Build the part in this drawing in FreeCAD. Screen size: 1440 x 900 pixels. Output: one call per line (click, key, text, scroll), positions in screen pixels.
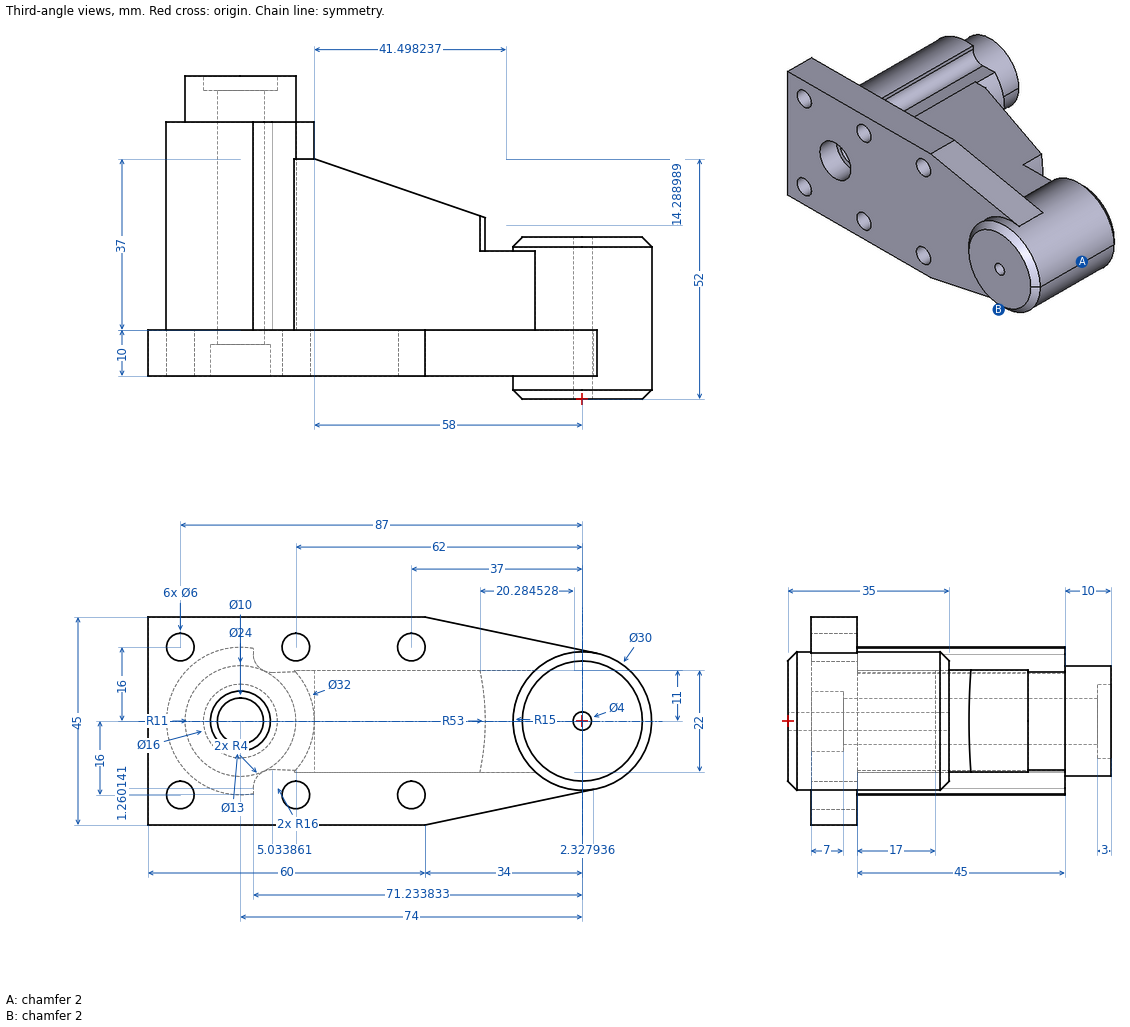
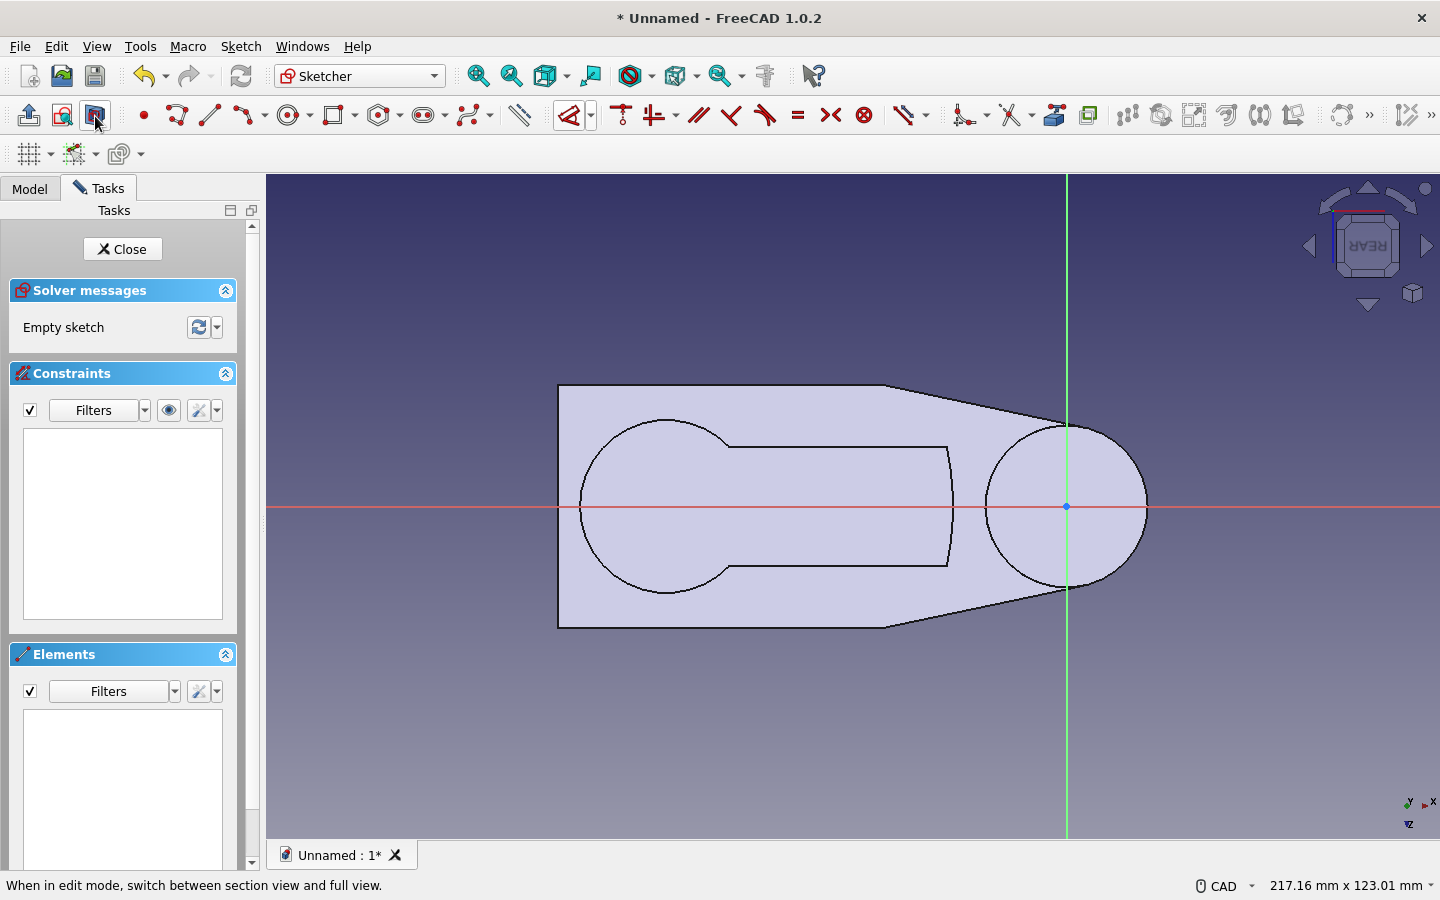
scroll(1102, 506, up, 6)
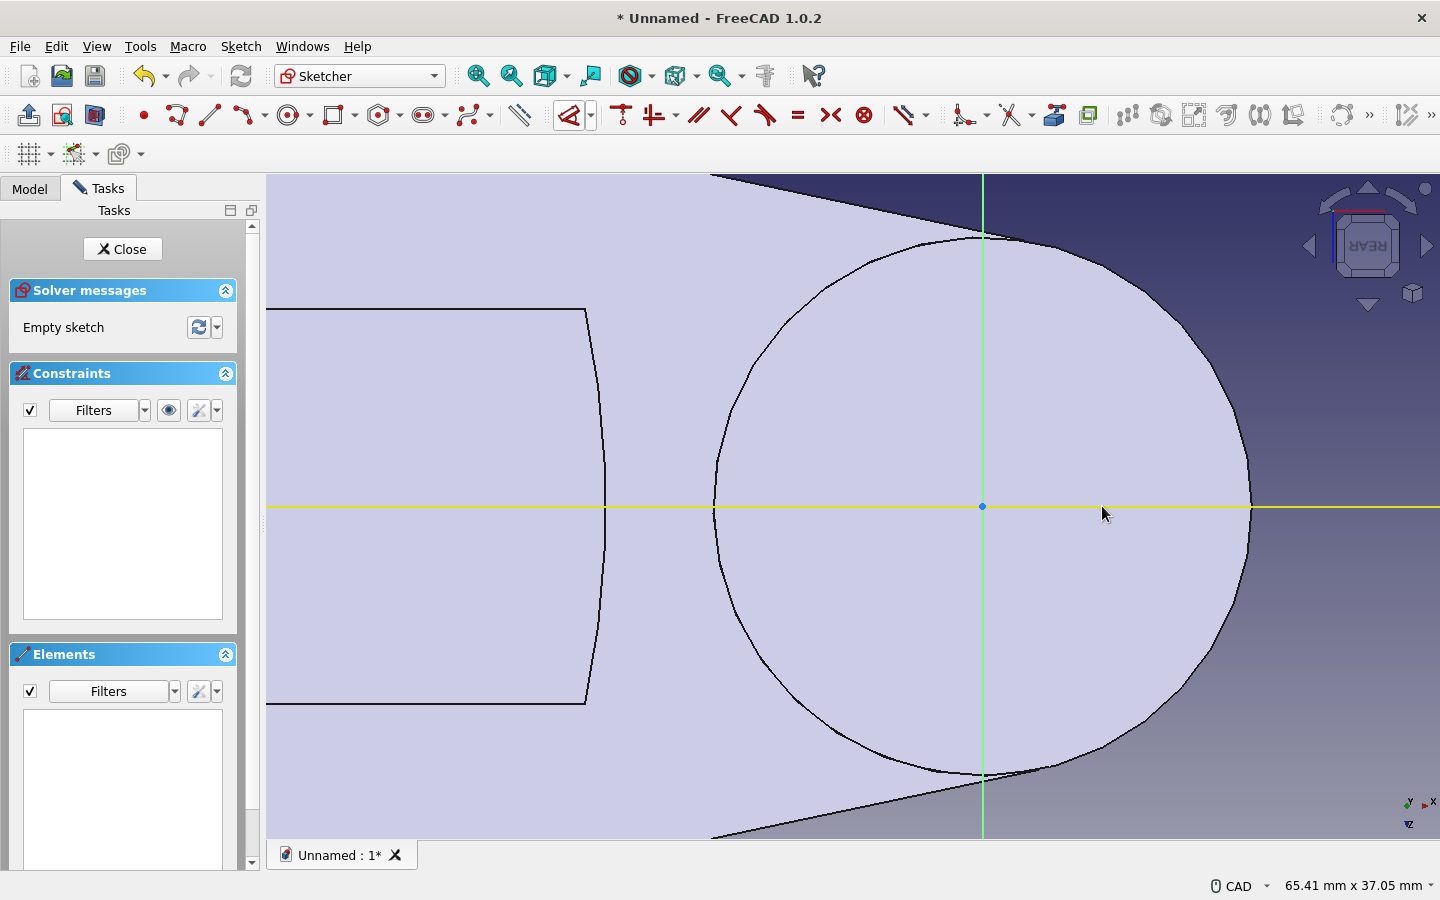
click(177, 116)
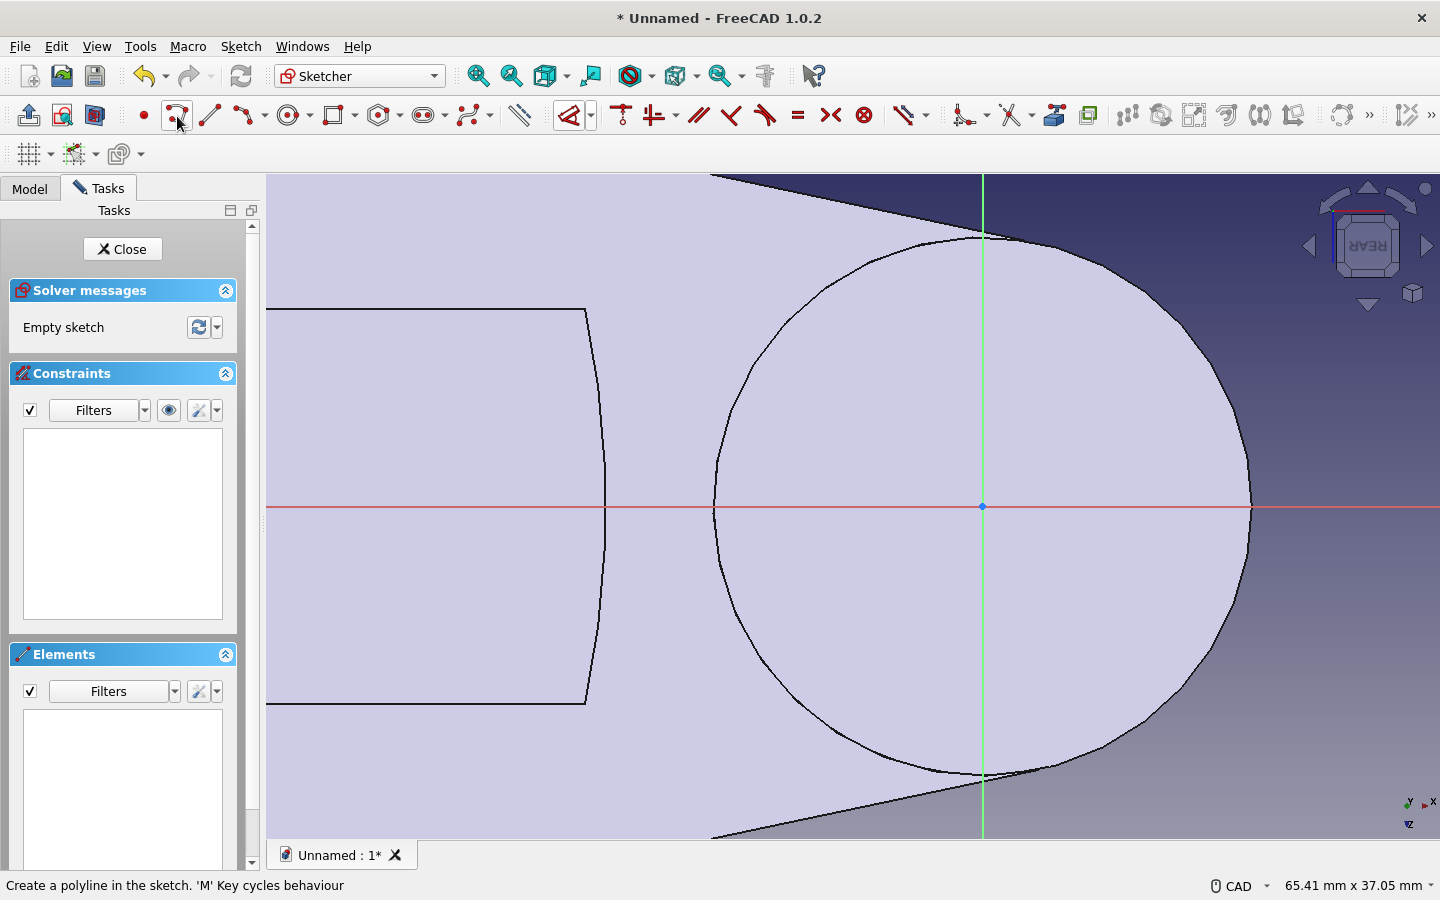
click(585, 704)
click(949, 704)
click(949, 309)
click(585, 309)
right_click(585, 309)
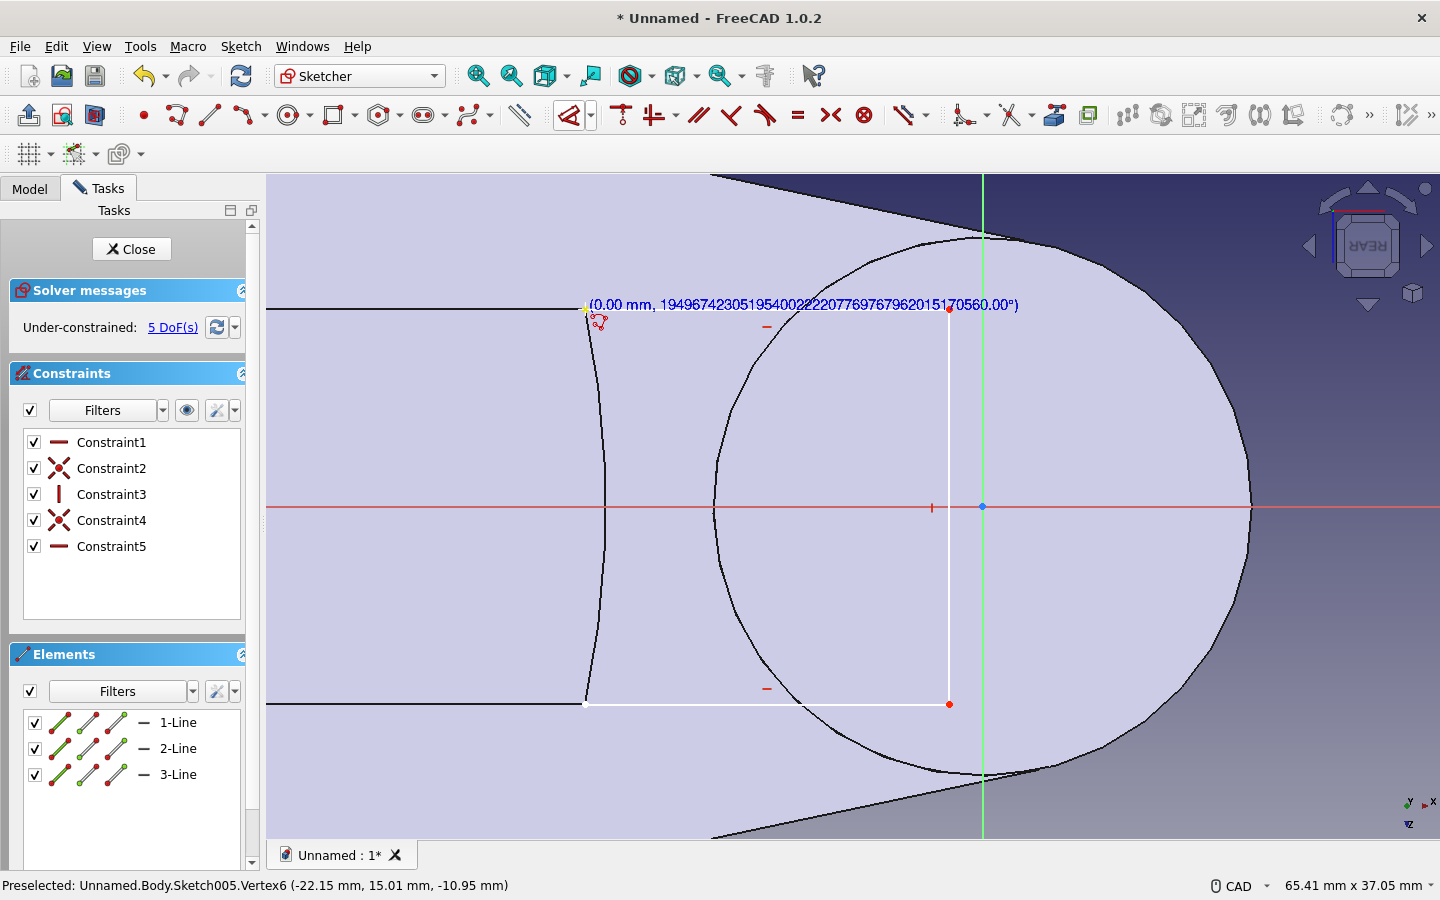
click(242, 116)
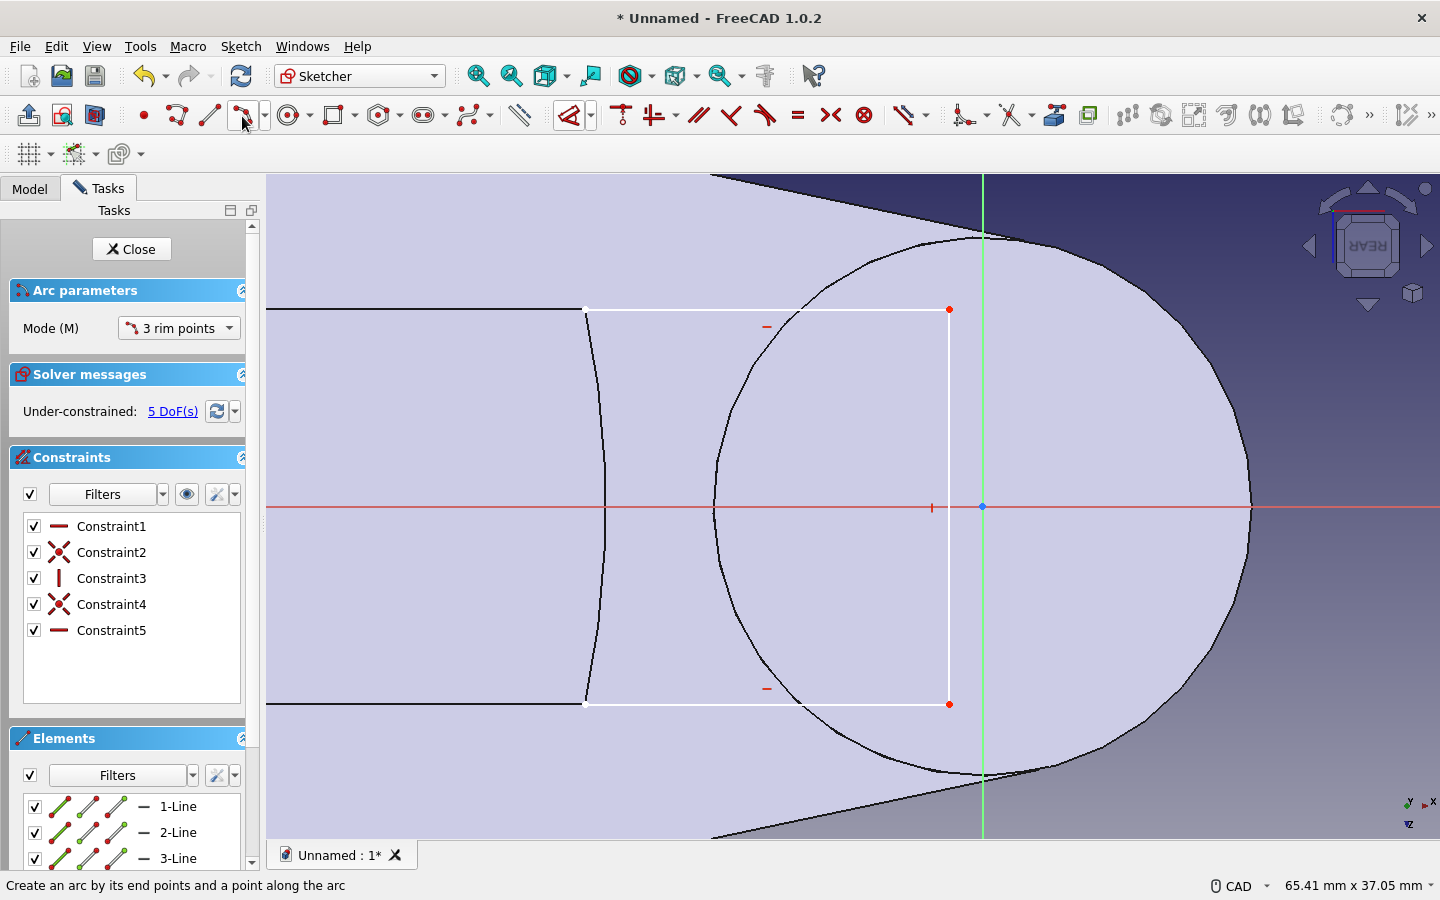
click(585, 310)
click(585, 705)
click(605, 546)
key(Escape)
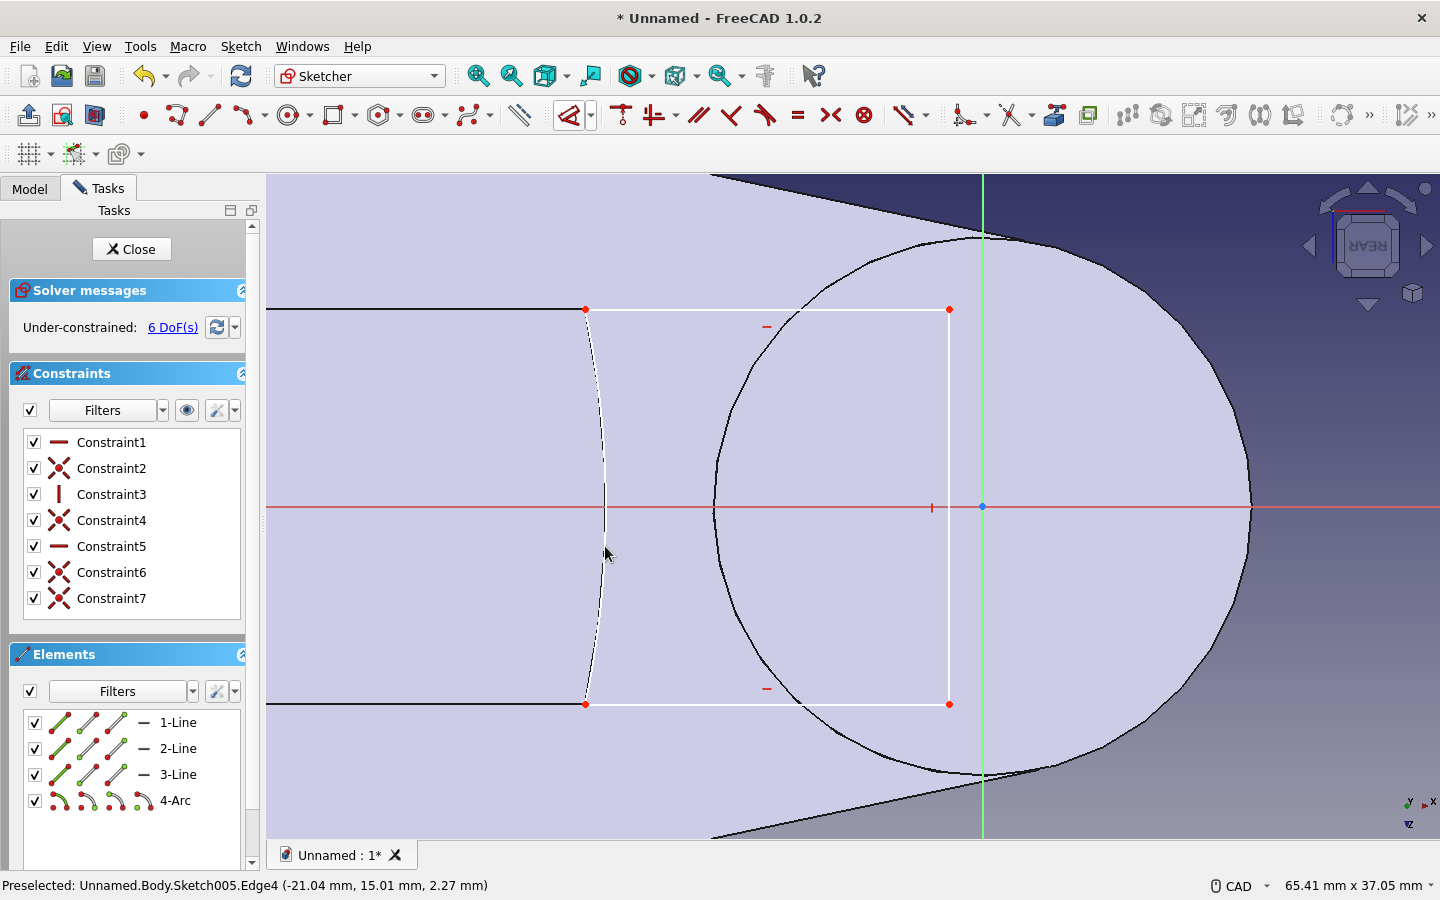
scroll(1275, 507, down, 3)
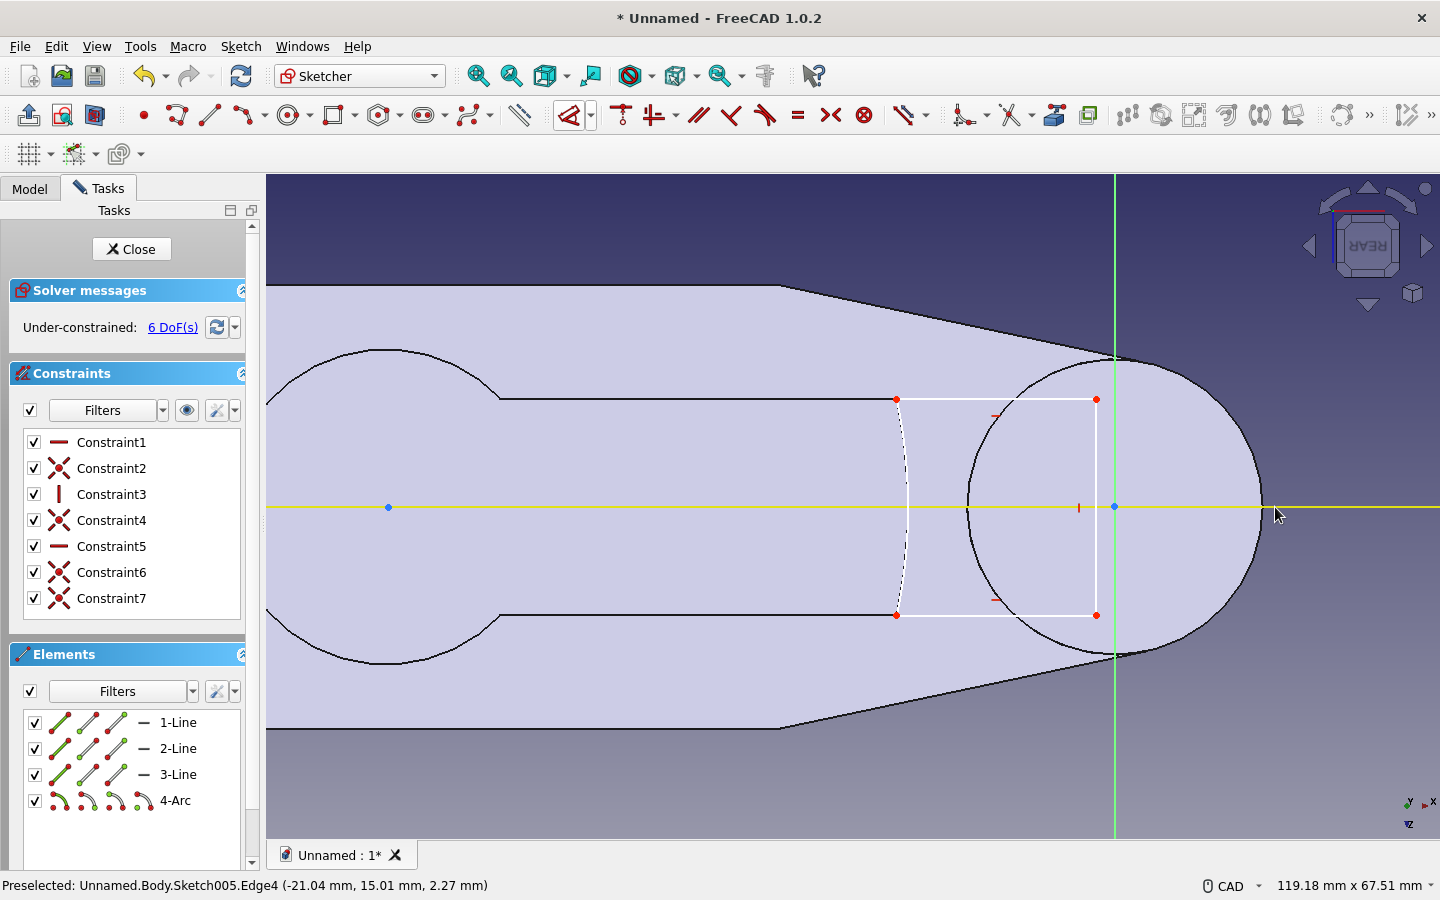
click(388, 508)